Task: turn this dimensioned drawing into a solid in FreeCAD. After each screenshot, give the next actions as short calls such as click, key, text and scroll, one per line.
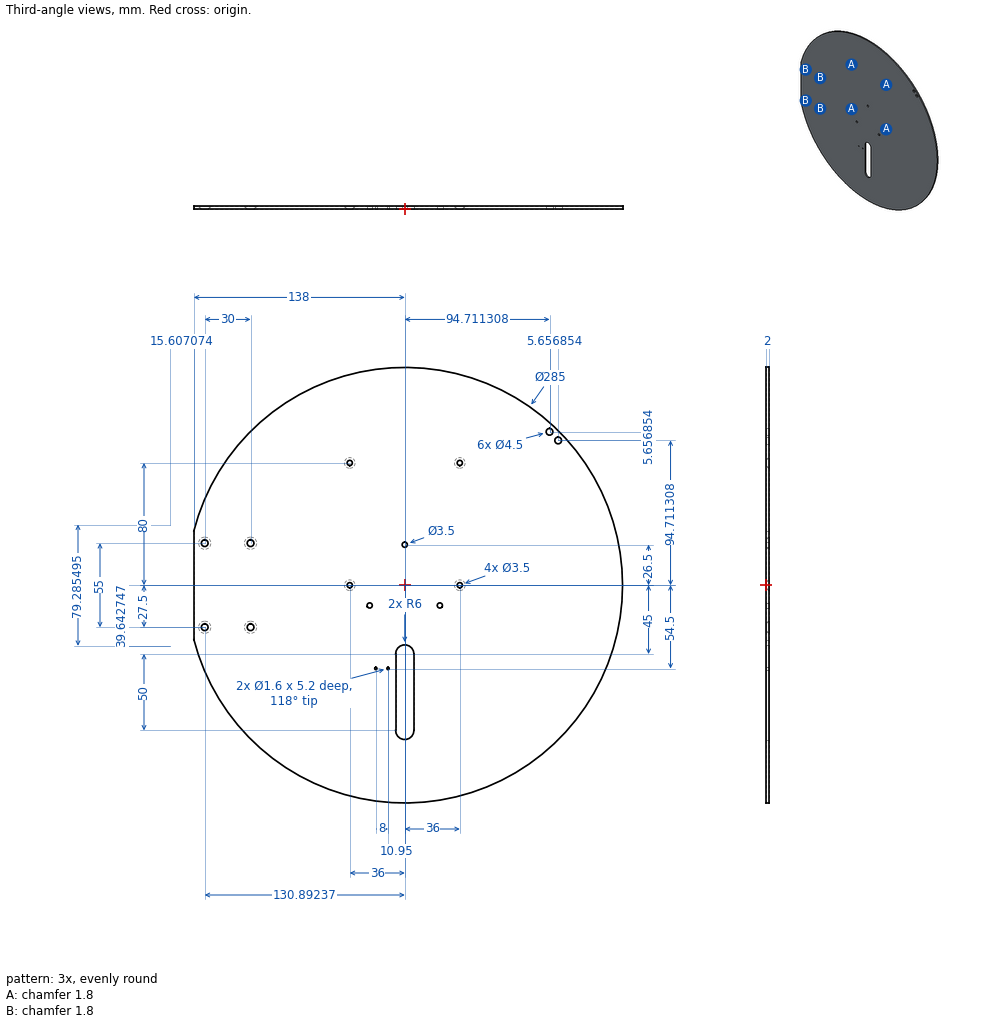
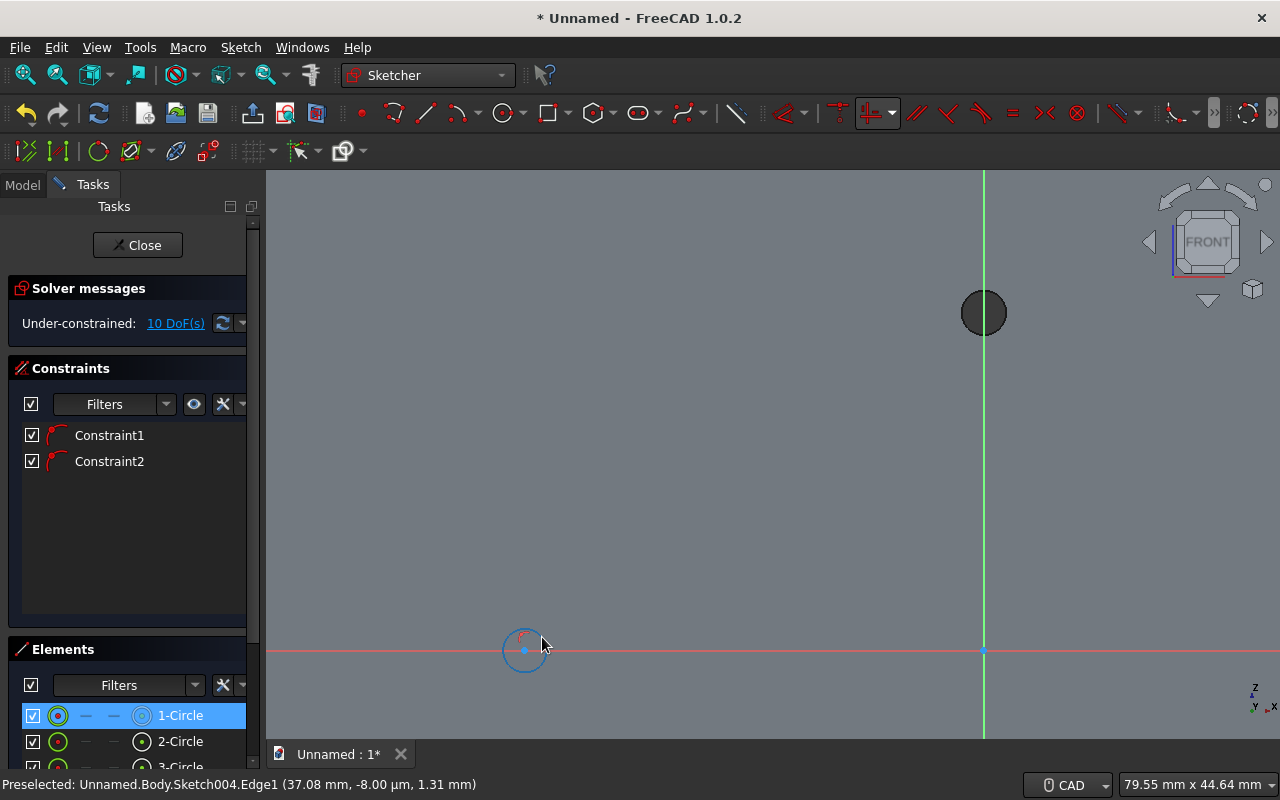
click(540, 635)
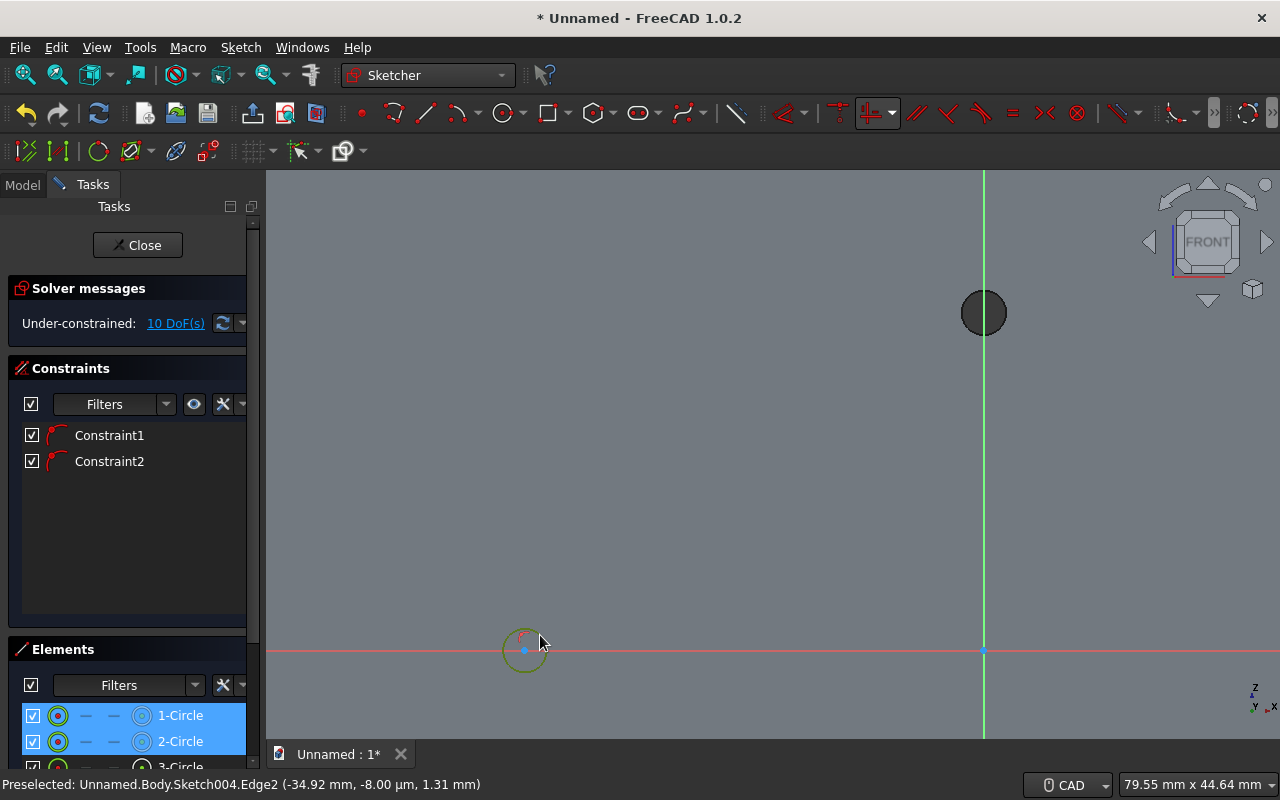
scroll(542, 637, down, 5)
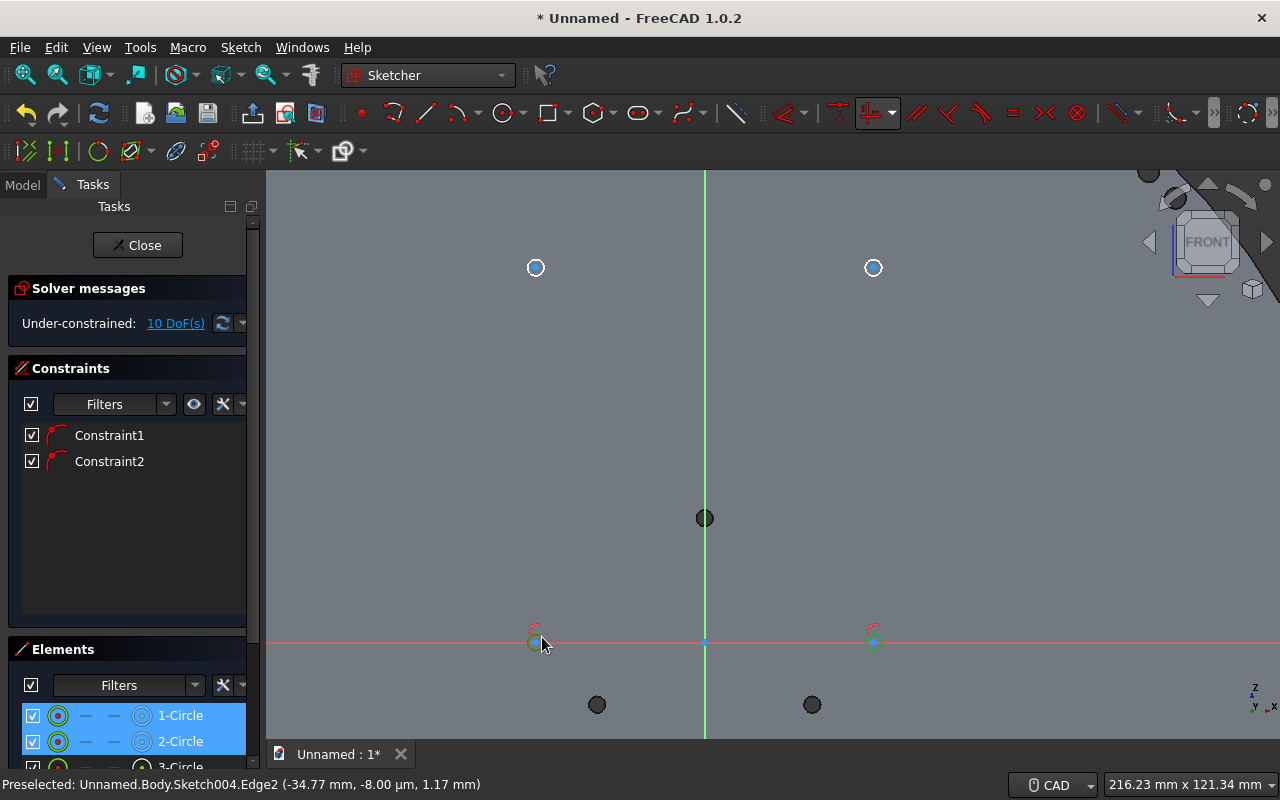
scroll(542, 262, up, 3)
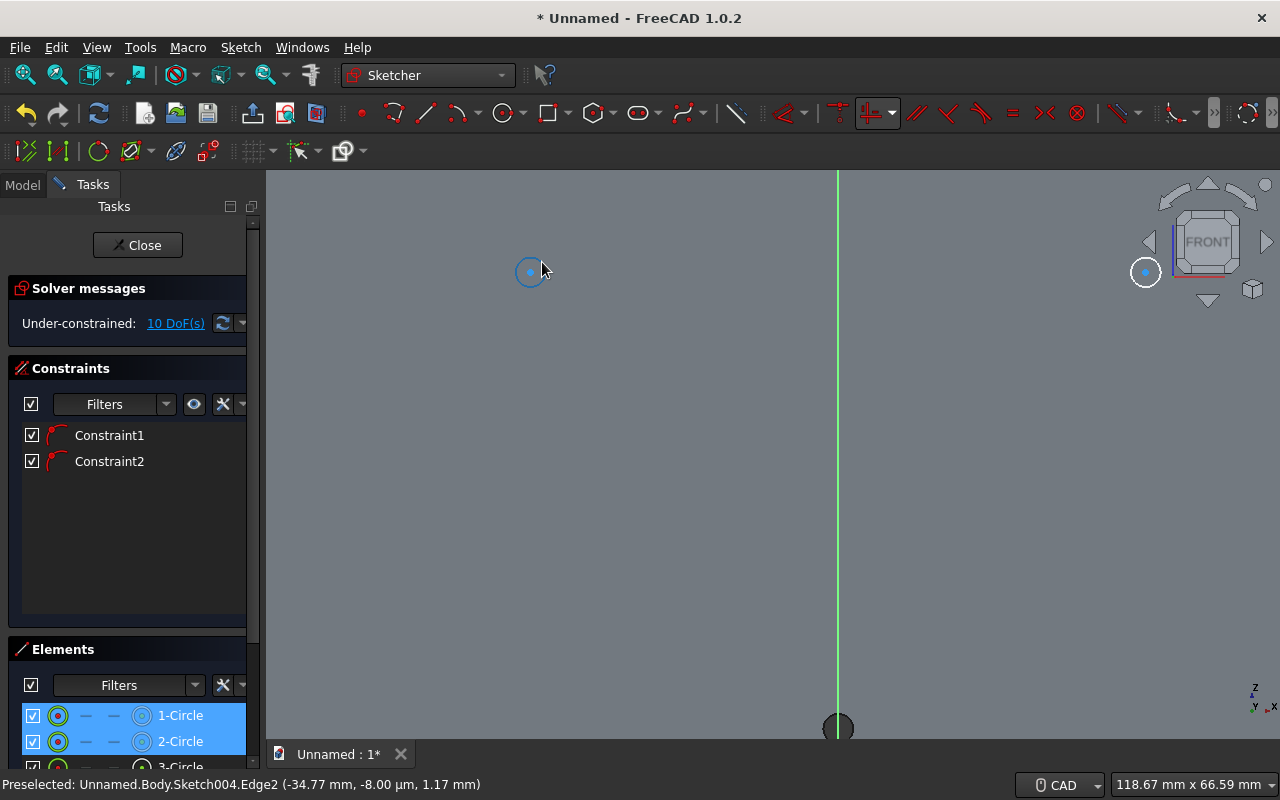
click(541, 262)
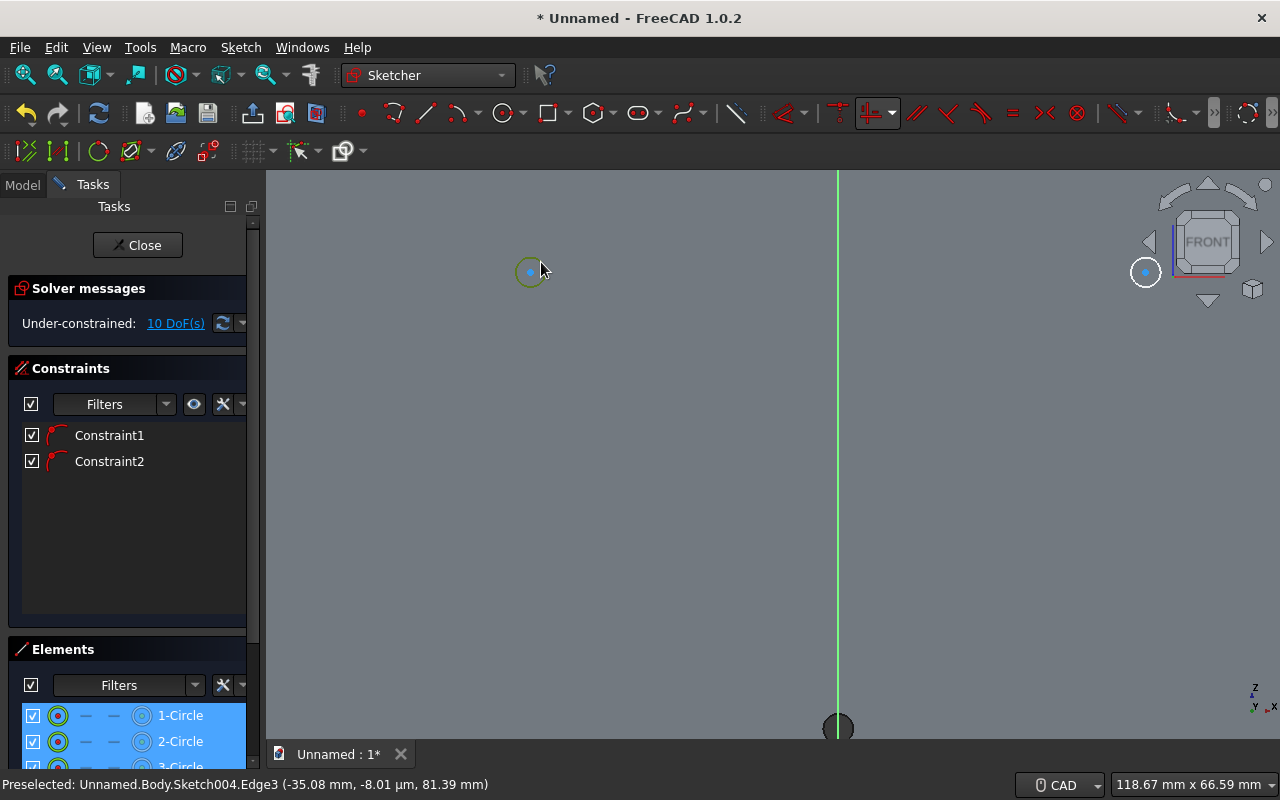
scroll(542, 261, down, 3)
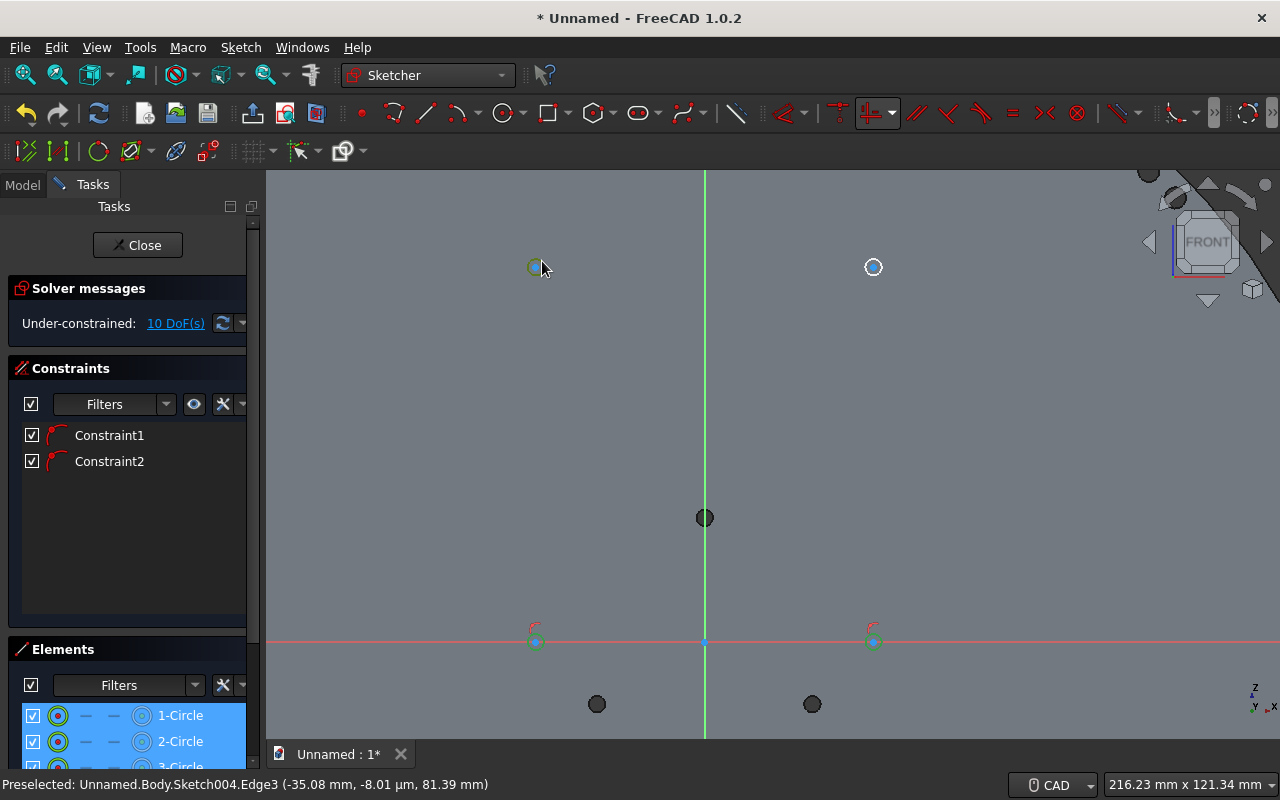
scroll(879, 262, up, 3)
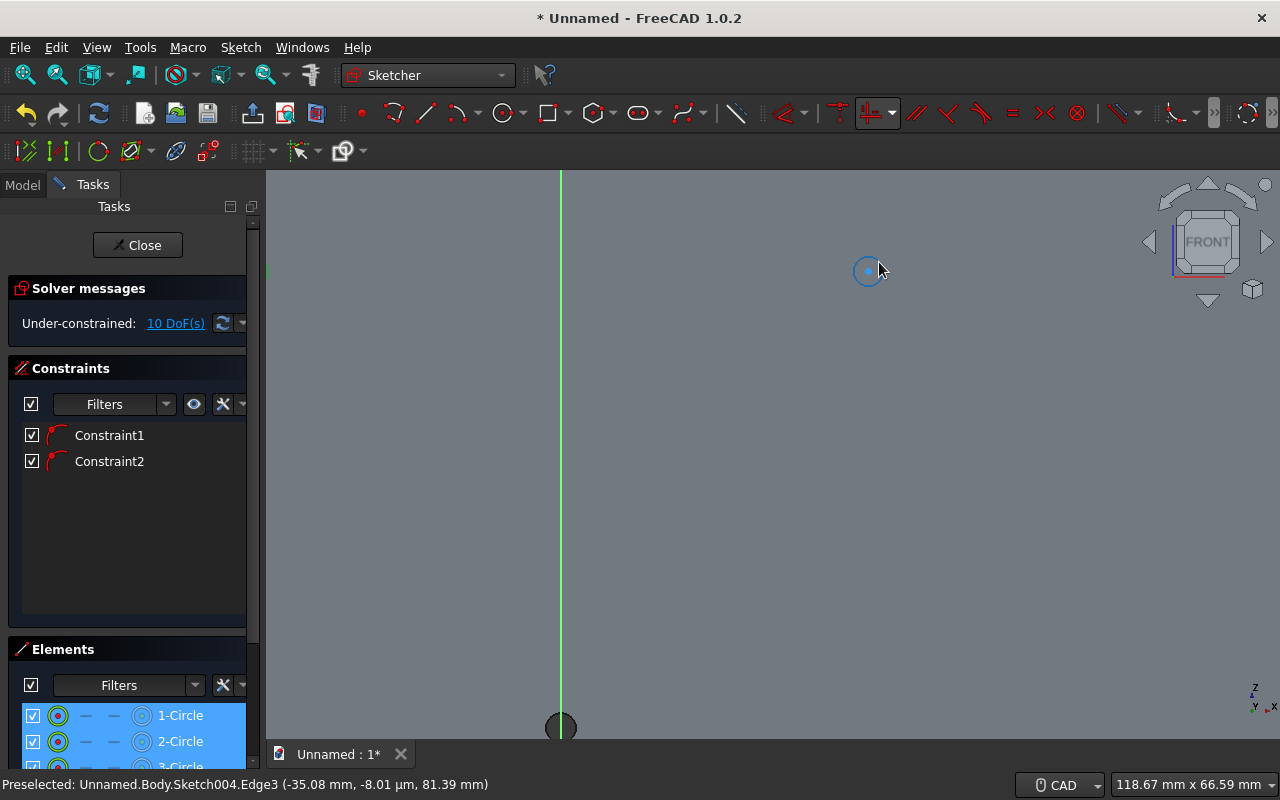
click(879, 261)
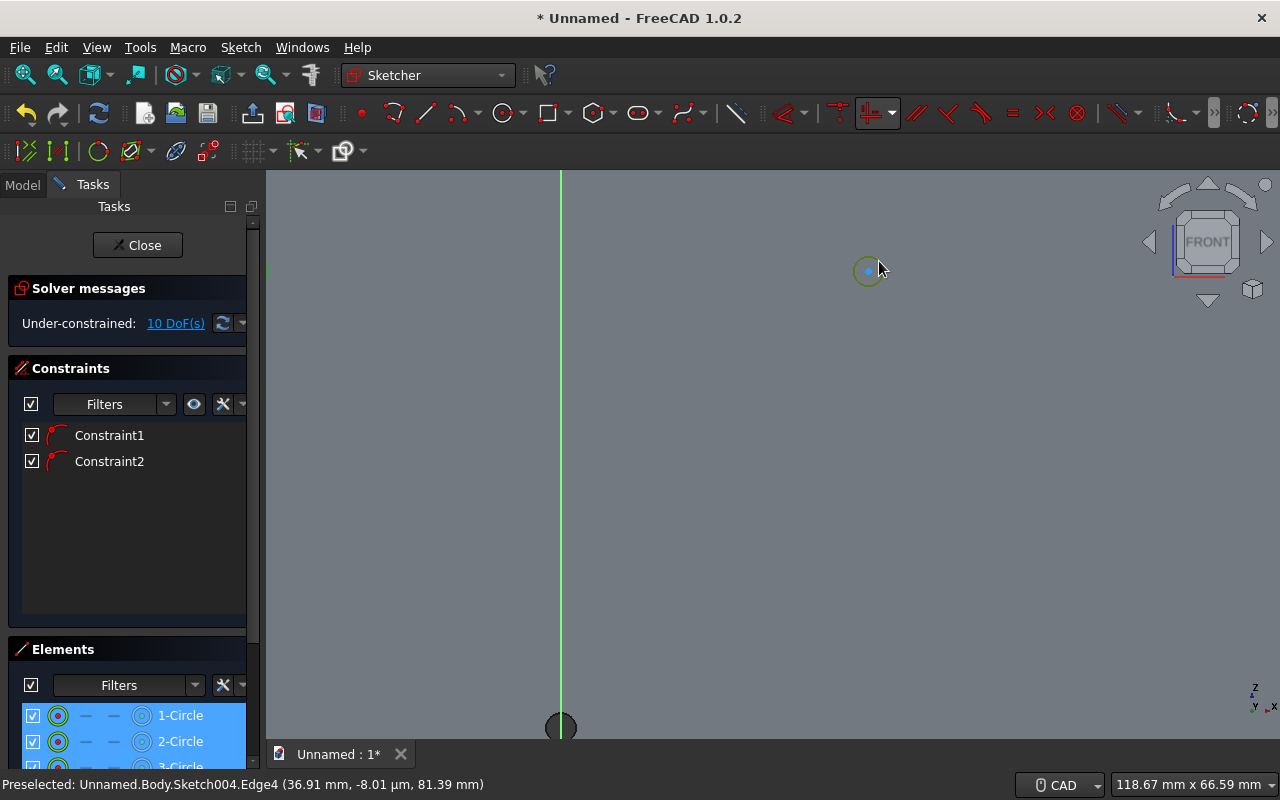
key(e)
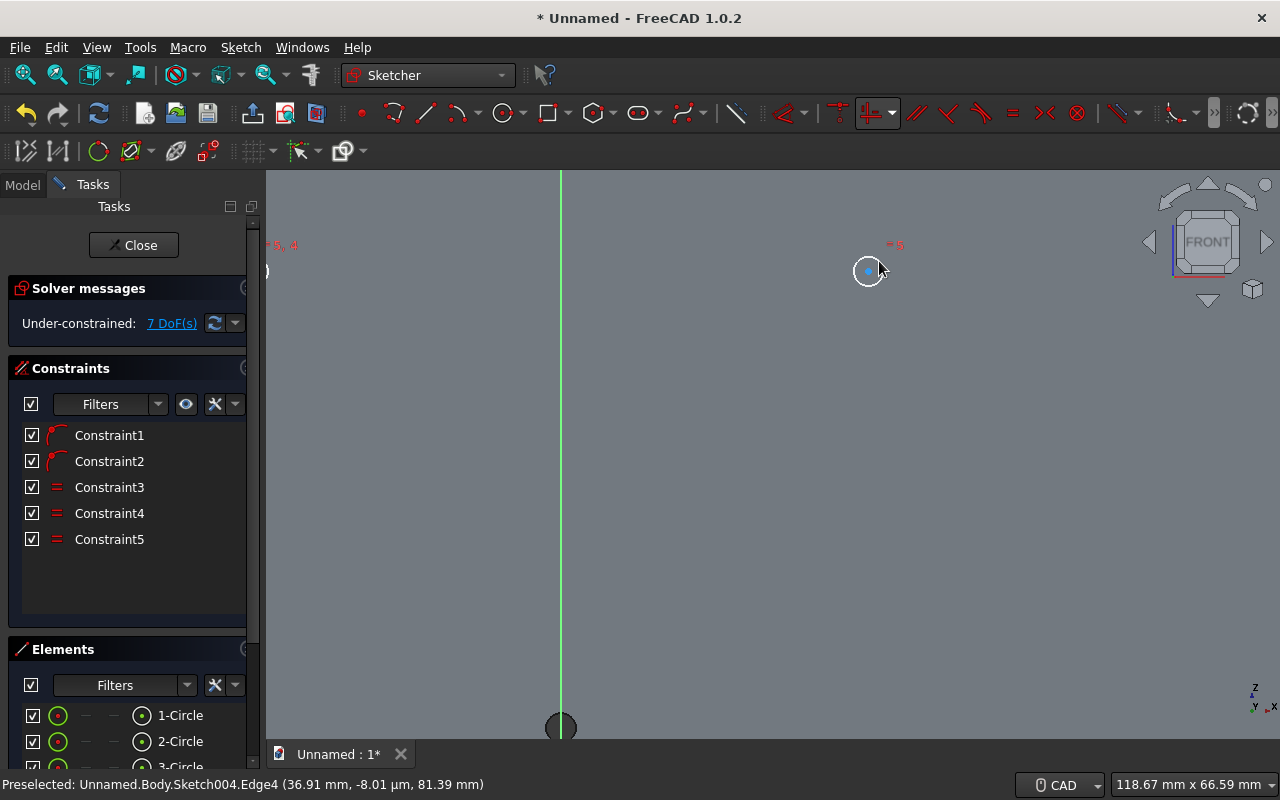
scroll(879, 262, down, 3)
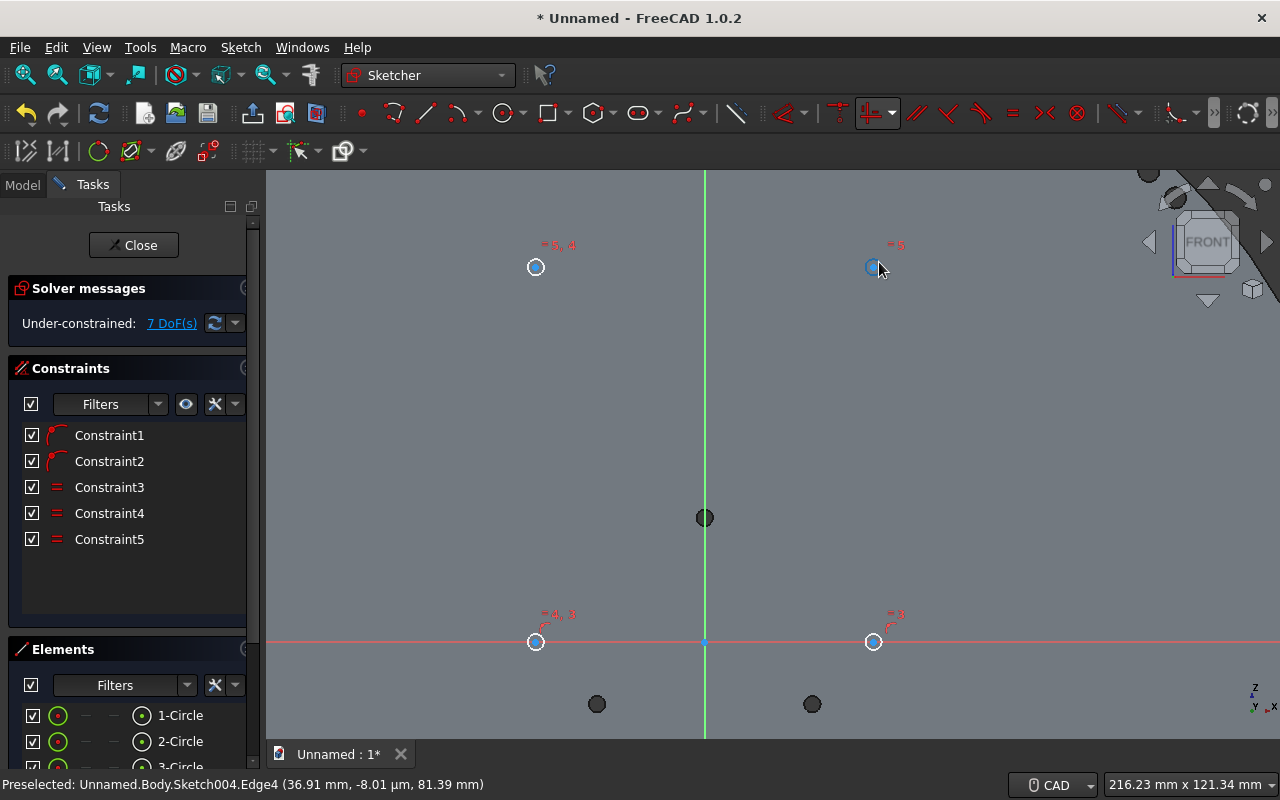
click(536, 642)